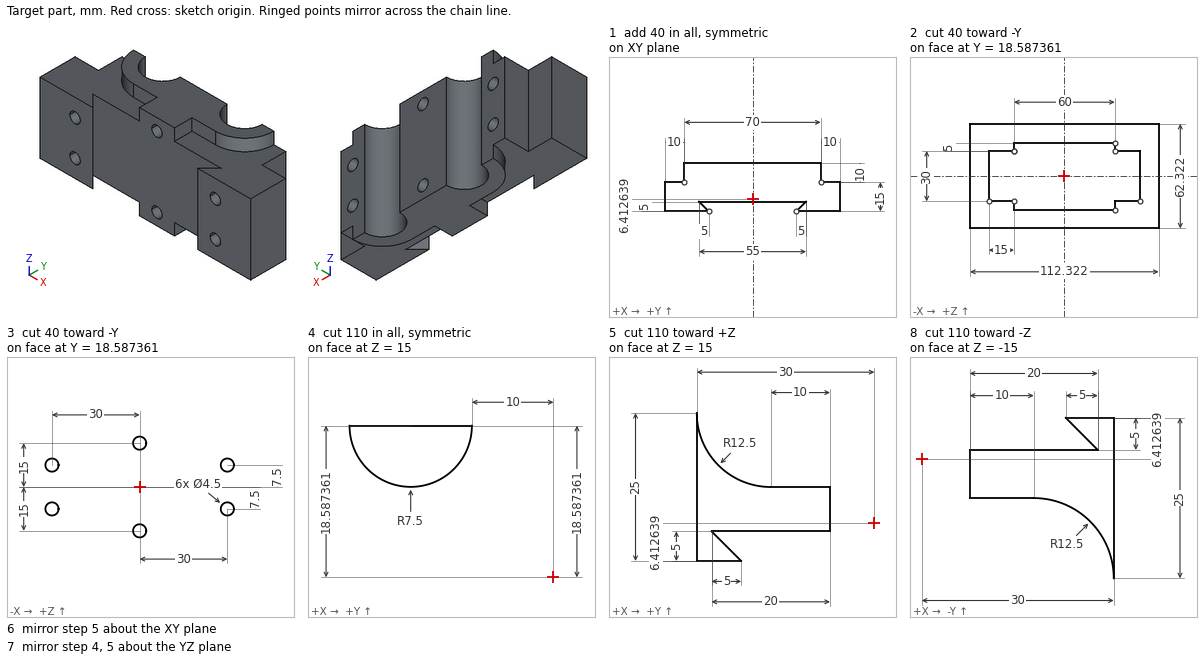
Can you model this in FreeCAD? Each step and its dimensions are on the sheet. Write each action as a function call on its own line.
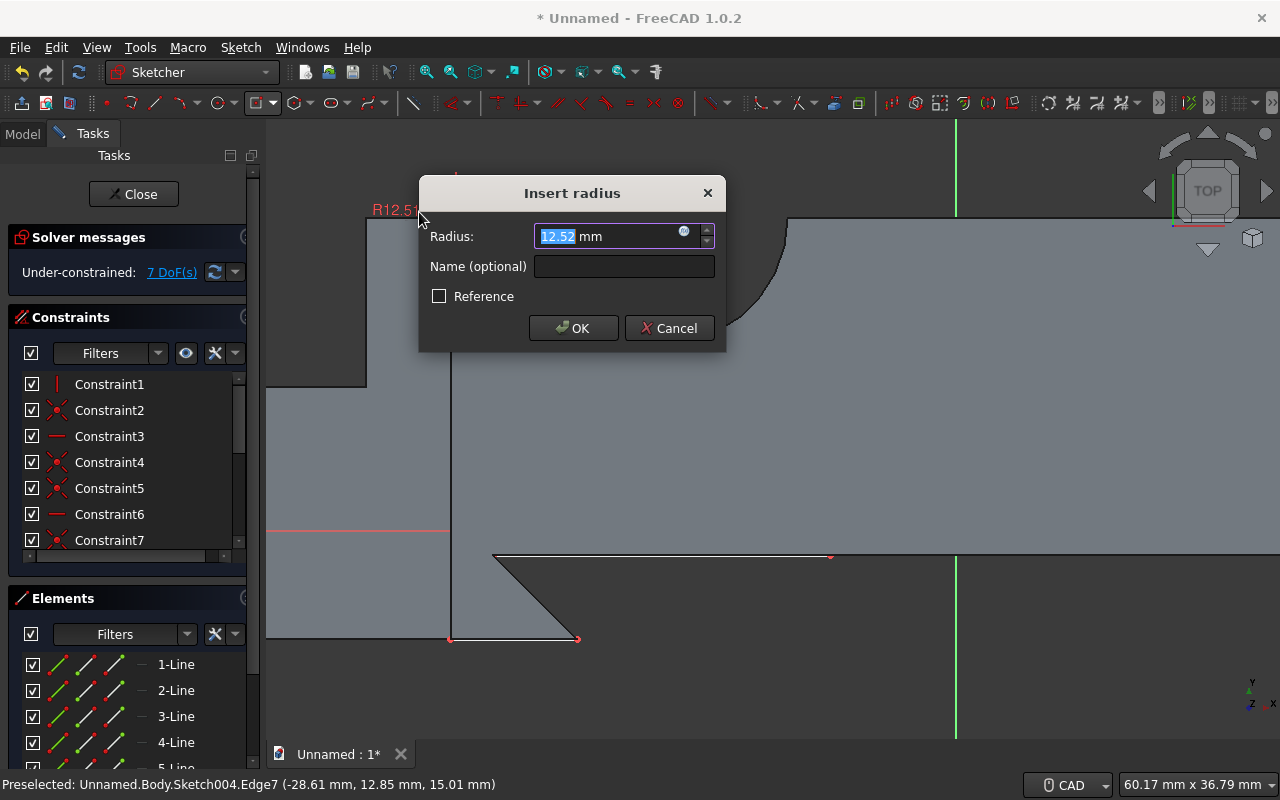
text(12.5)
key(Return)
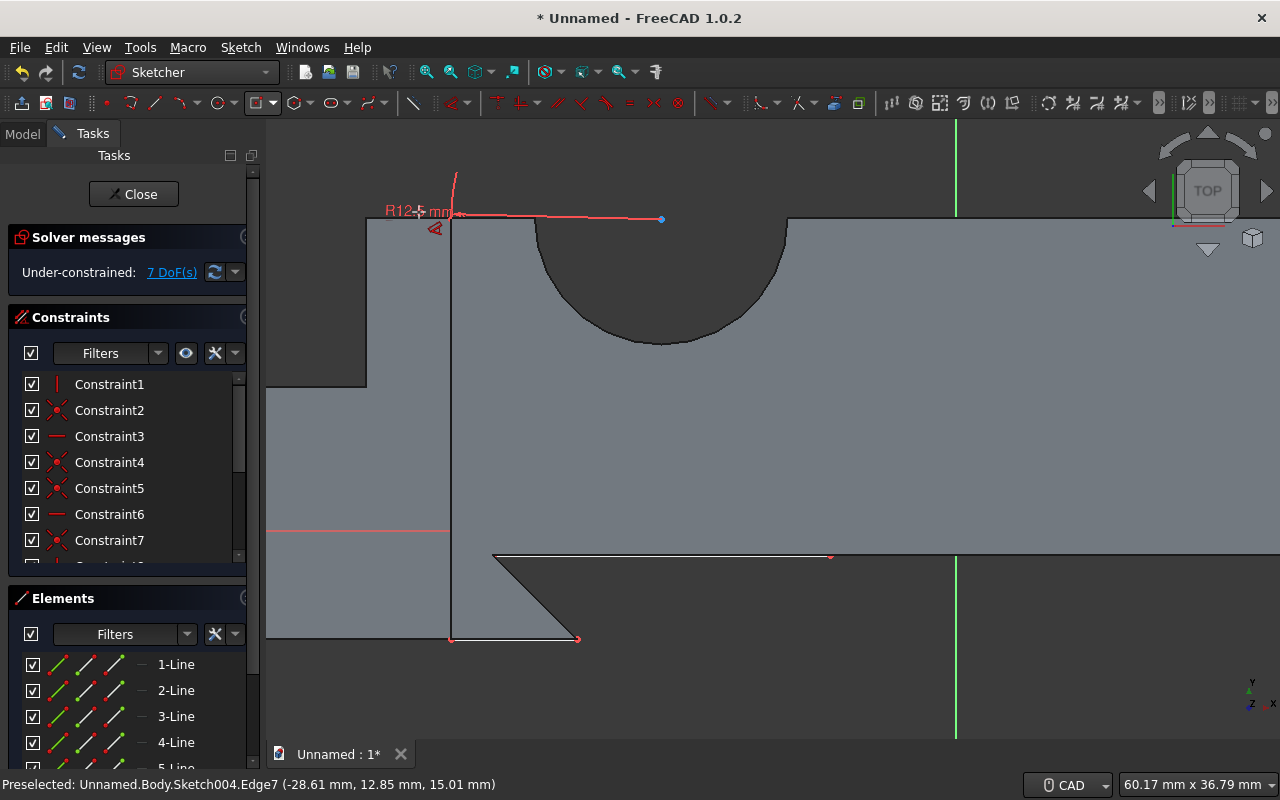
click(451, 346)
click(417, 430)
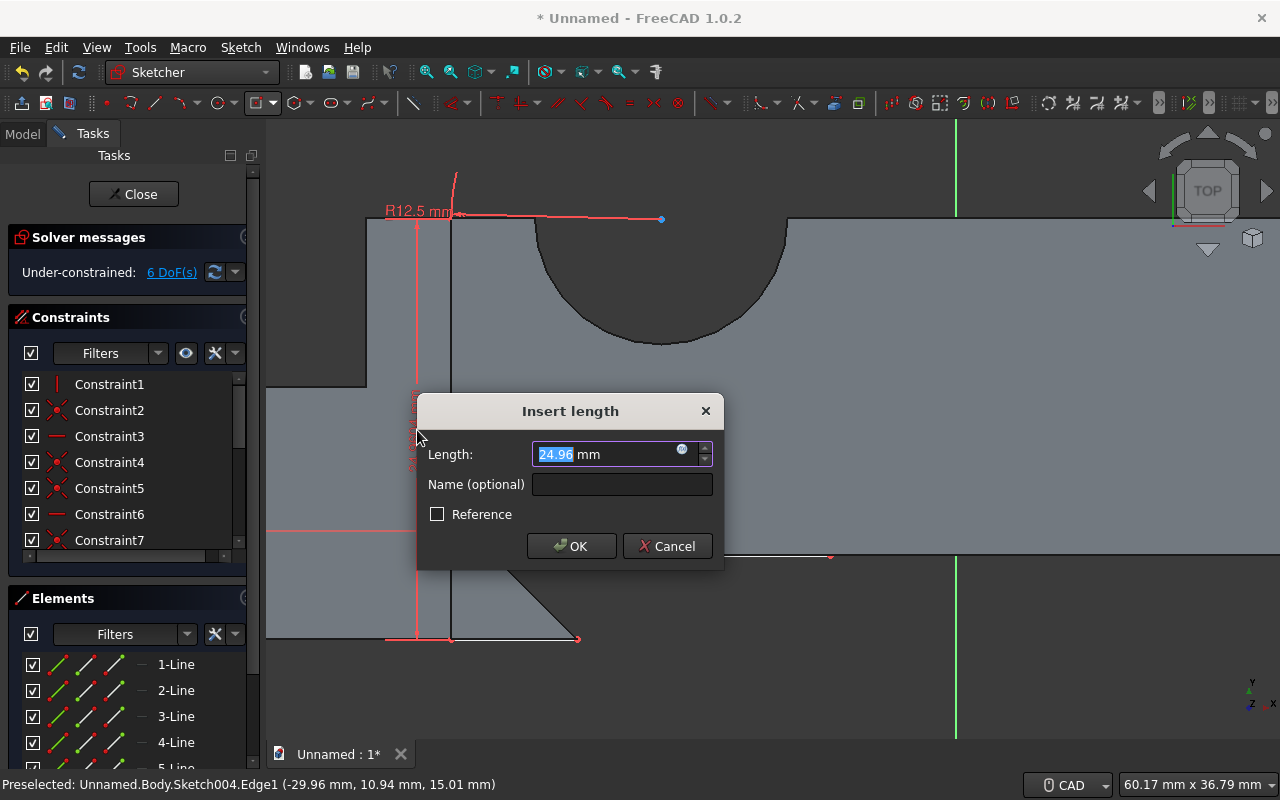
text(25)
key(Return)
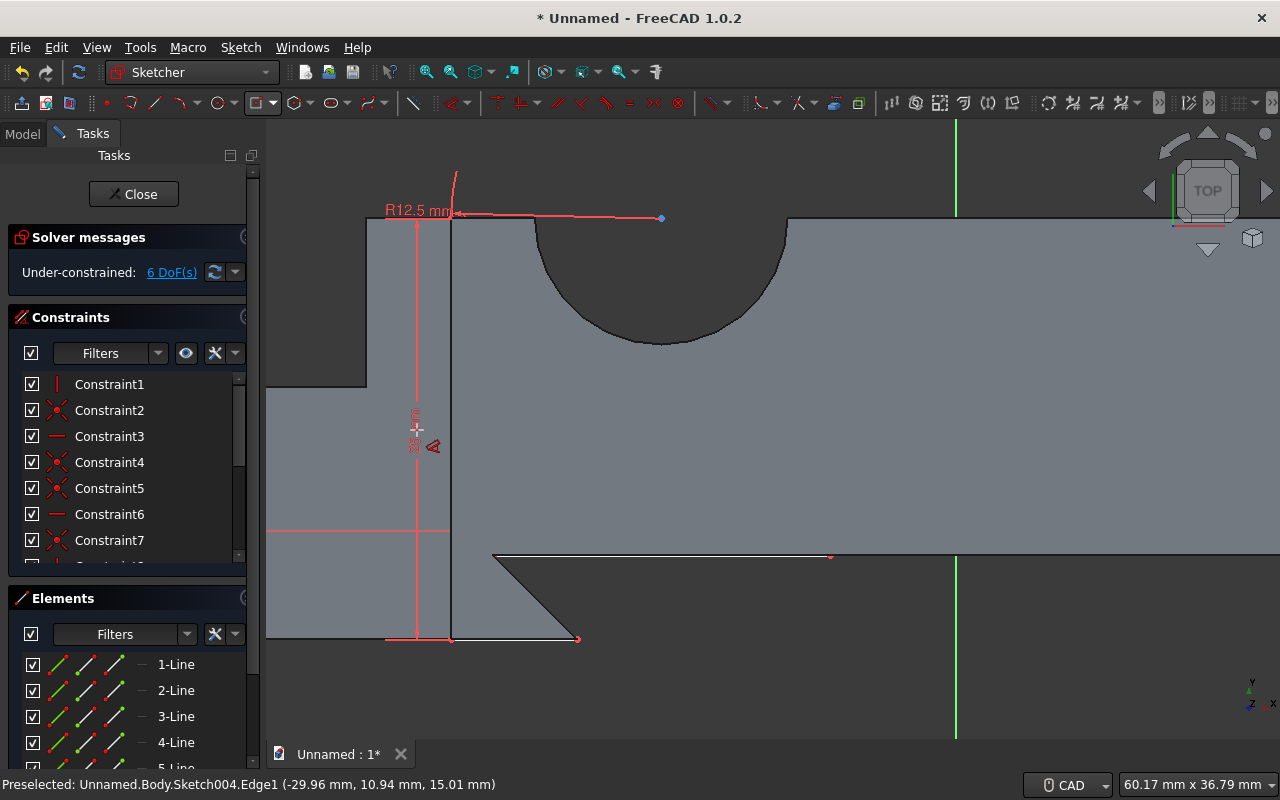
click(594, 556)
click(662, 590)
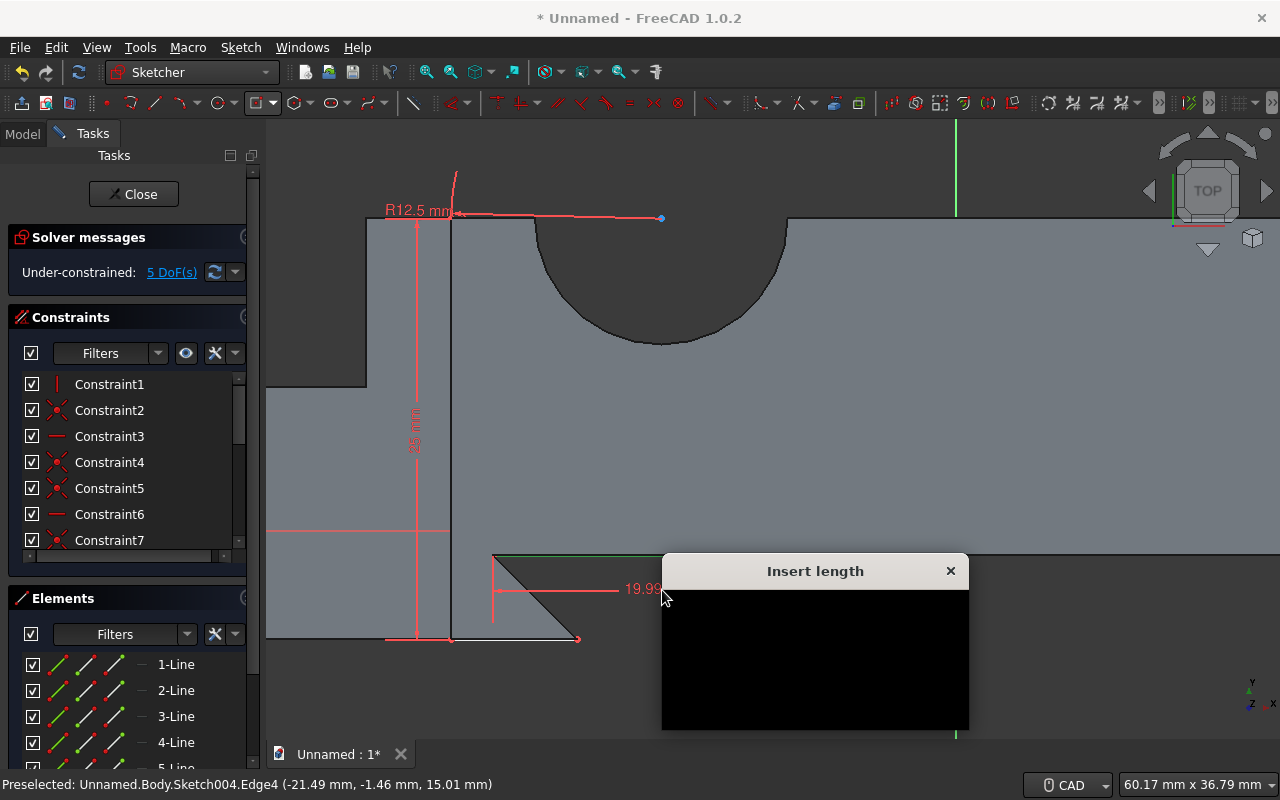
text(20)
key(Return)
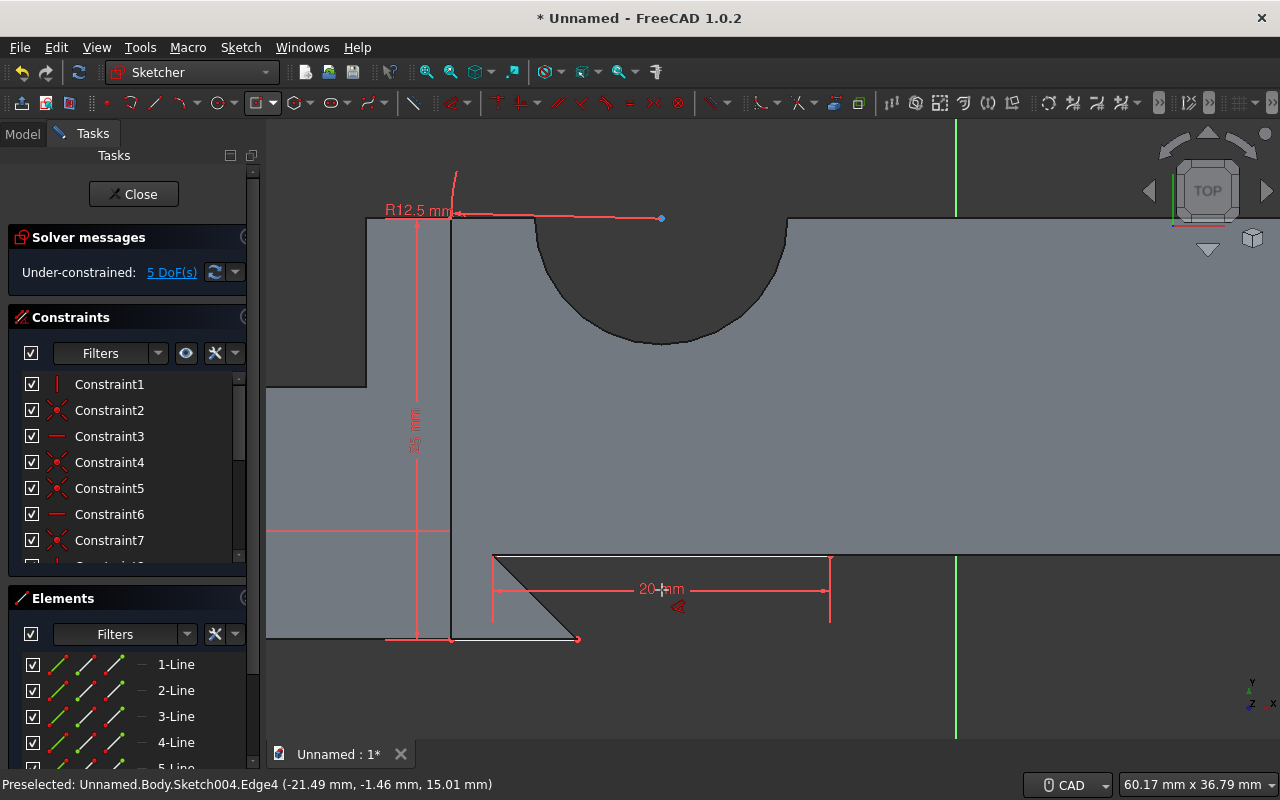
click(780, 429)
click(746, 463)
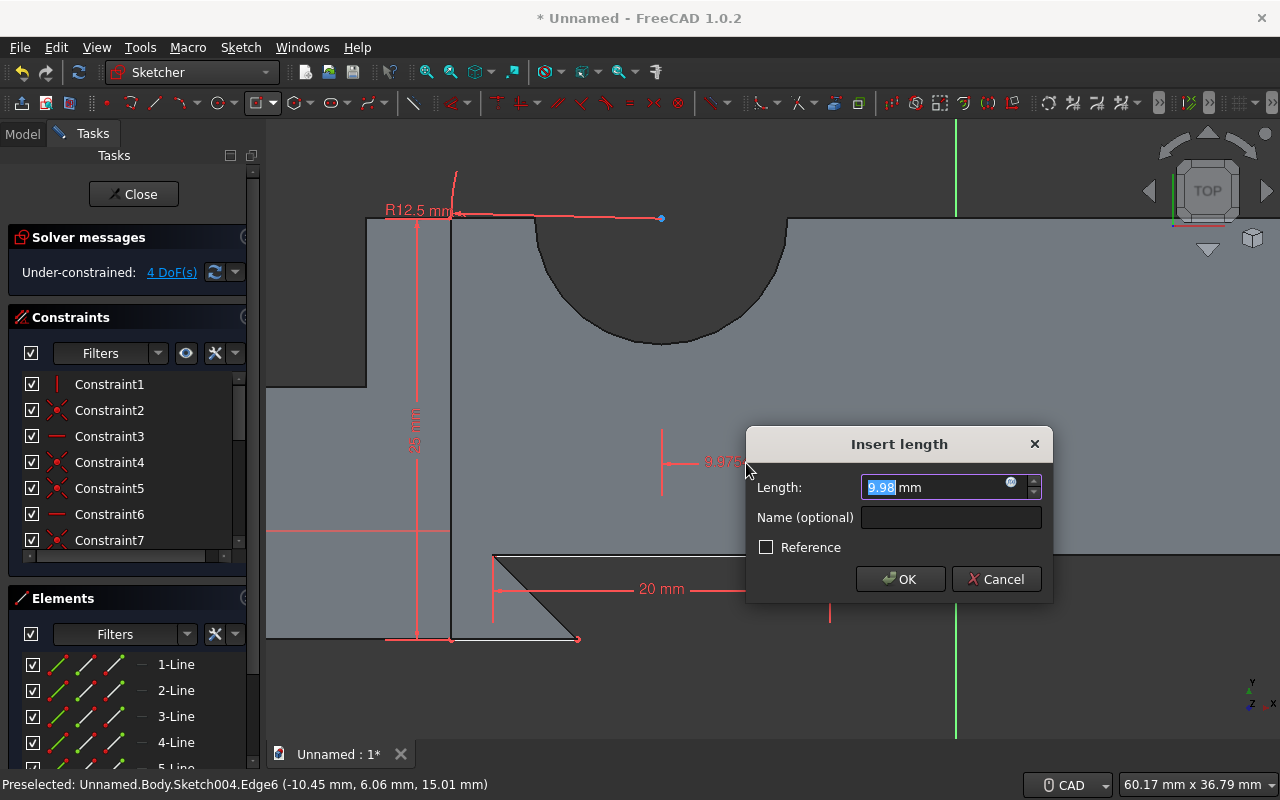
text(10)
key(Return)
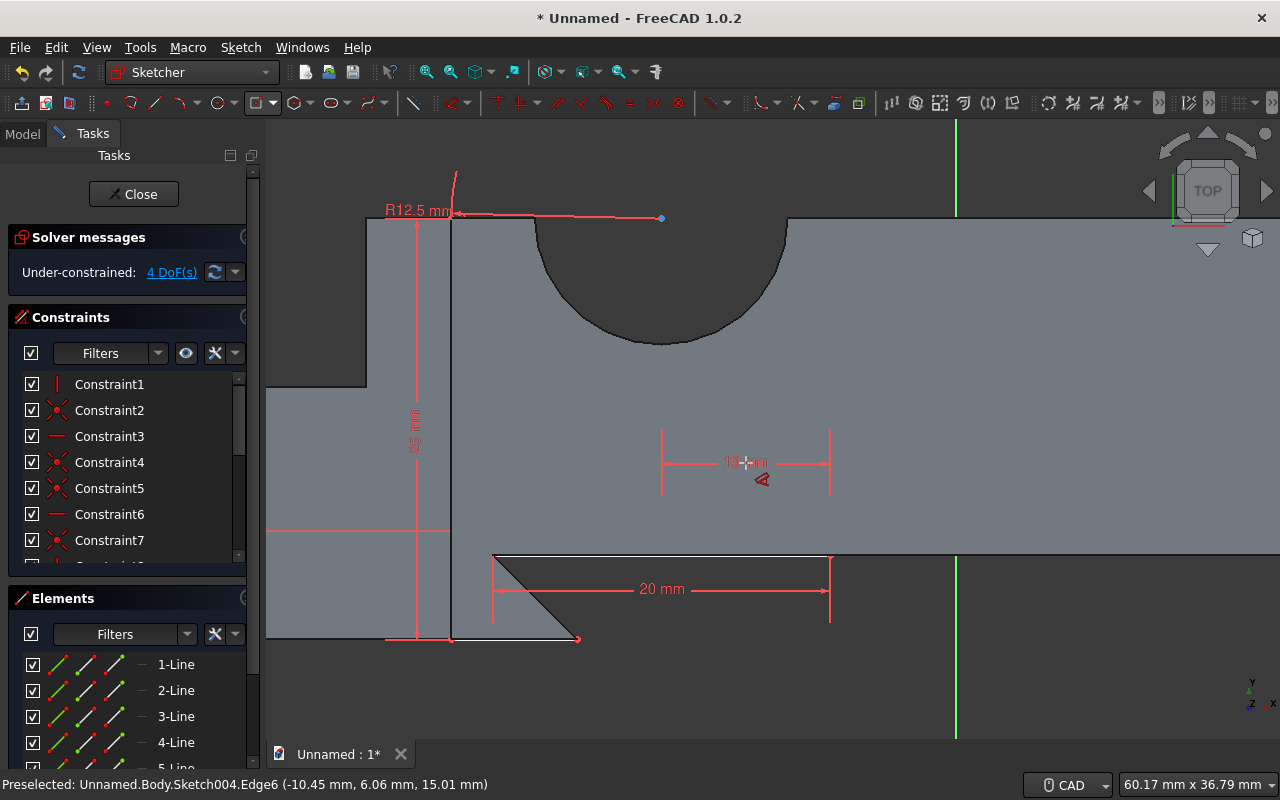
click(552, 615)
click(535, 674)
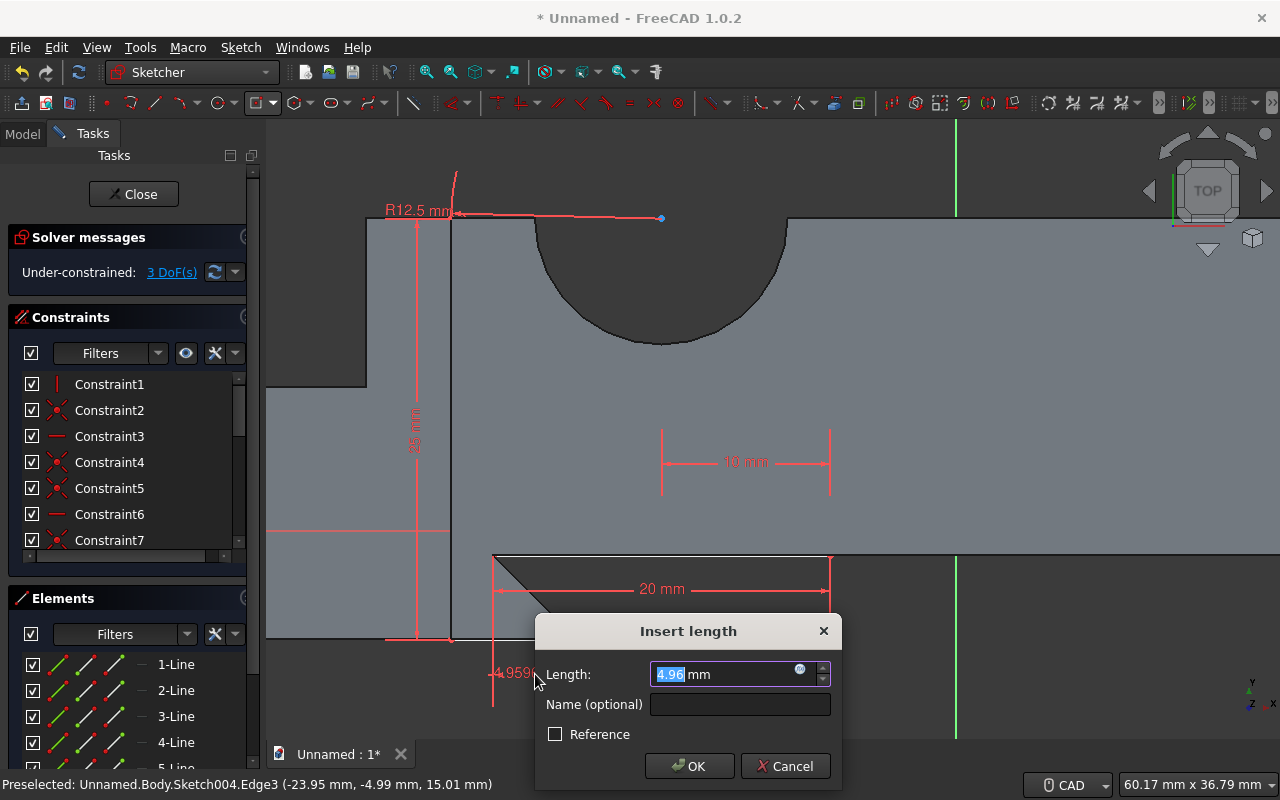
text(5)
key(Return)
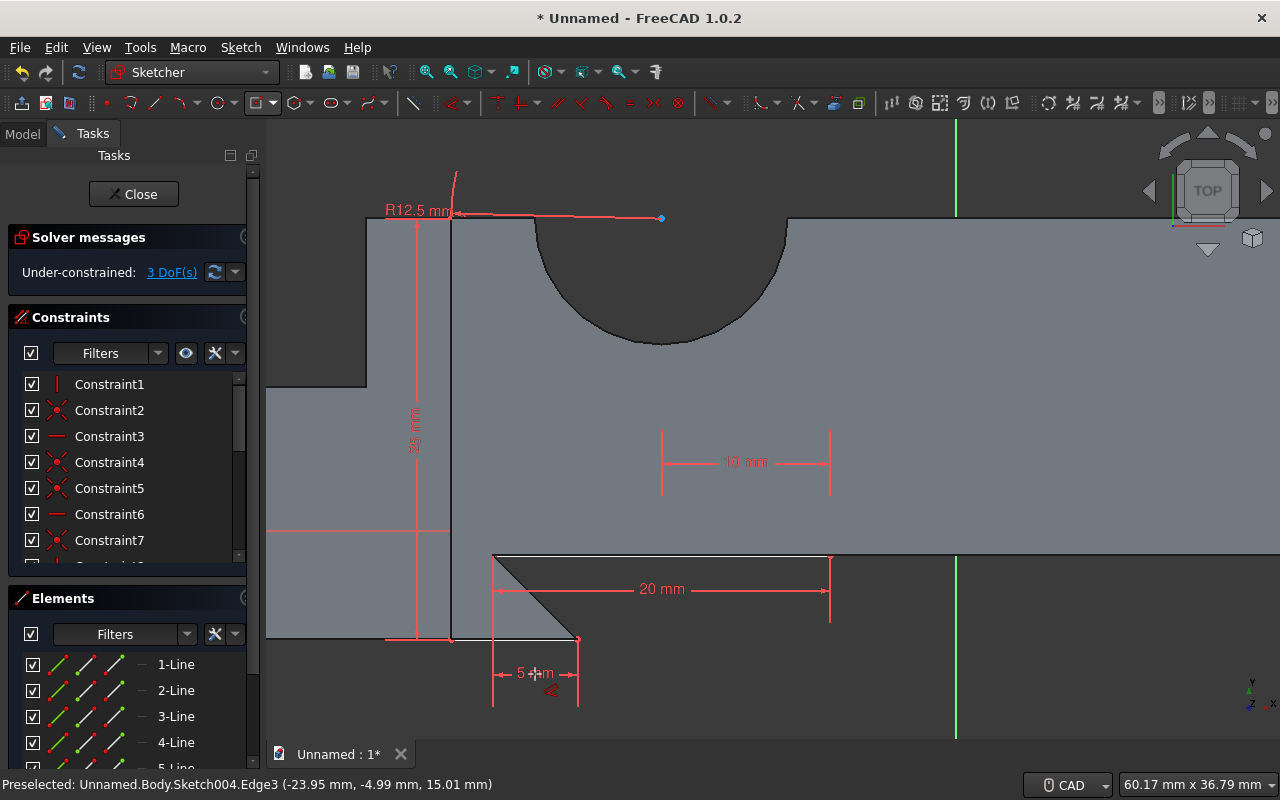
click(552, 615)
click(612, 617)